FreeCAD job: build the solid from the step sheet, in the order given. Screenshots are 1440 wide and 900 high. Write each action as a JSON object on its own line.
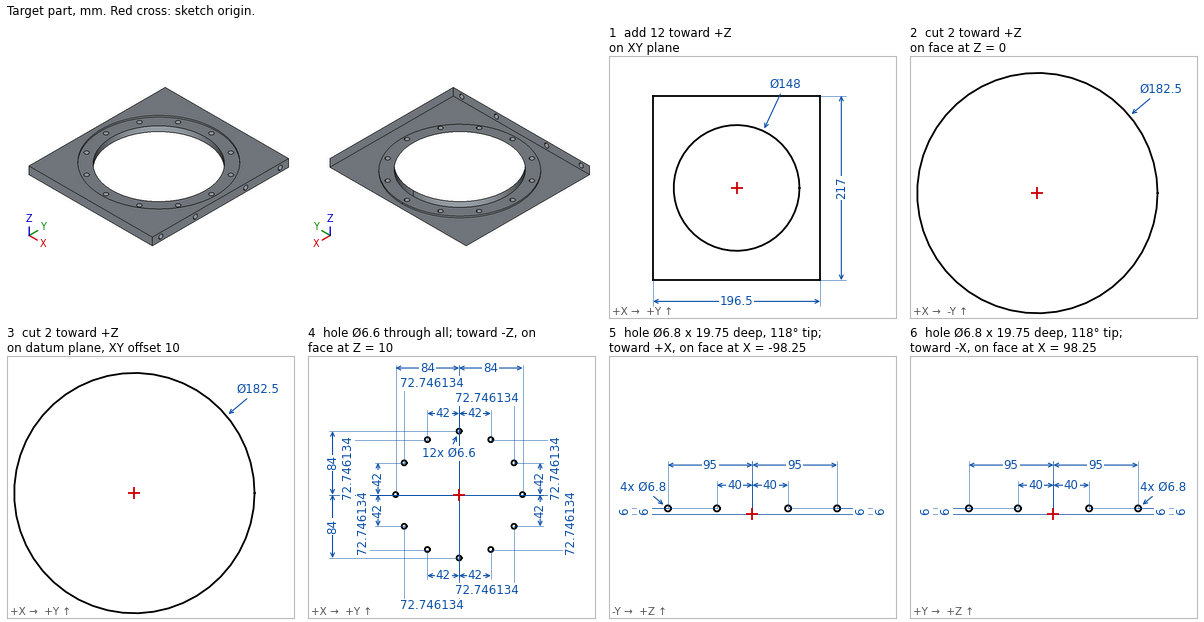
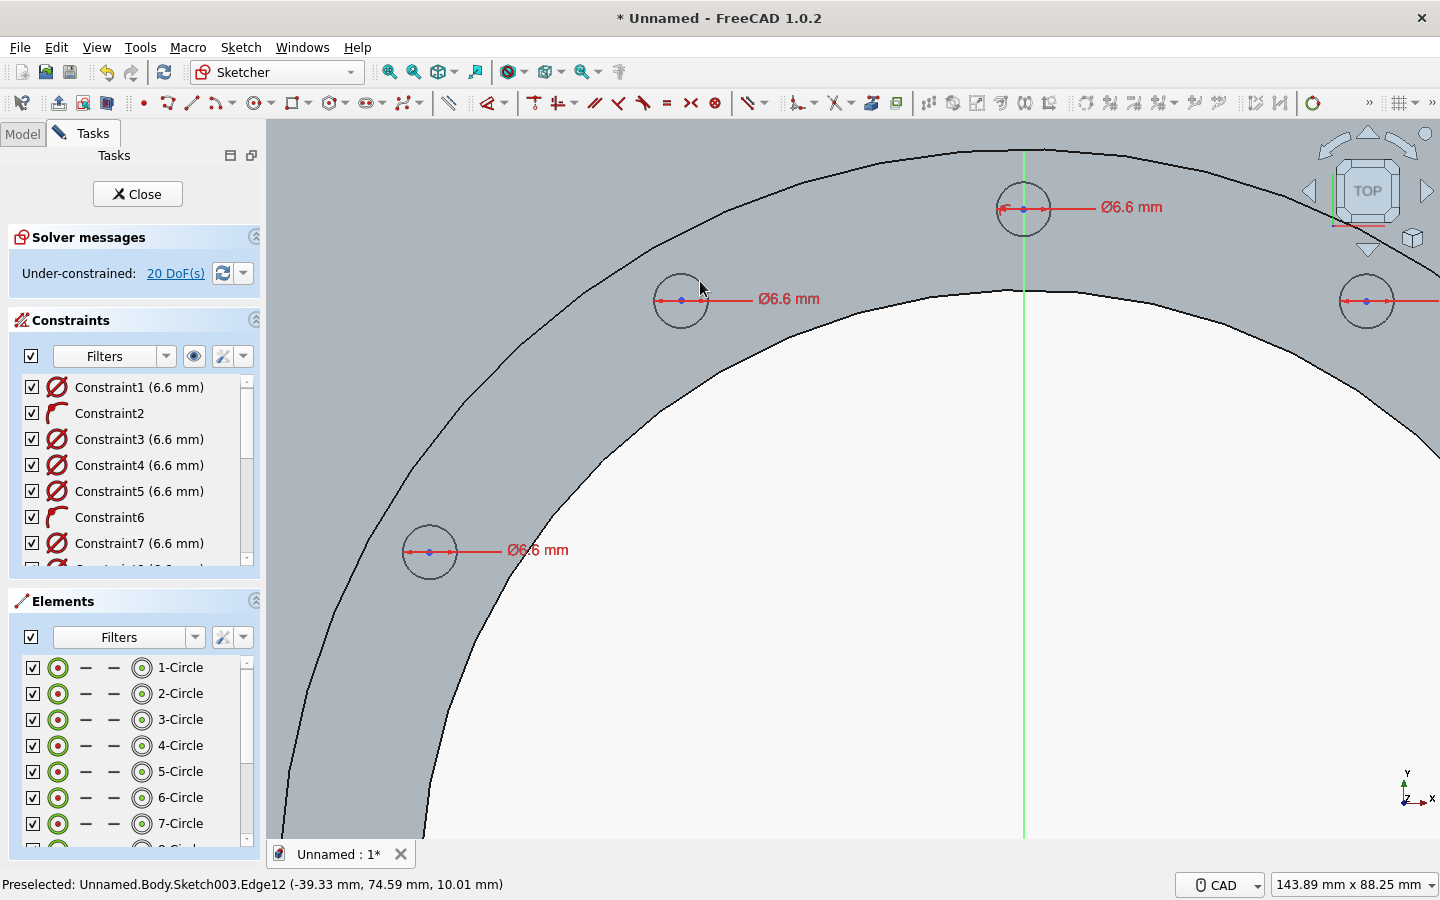
{"action": "left_click", "coordinate": [488, 104]}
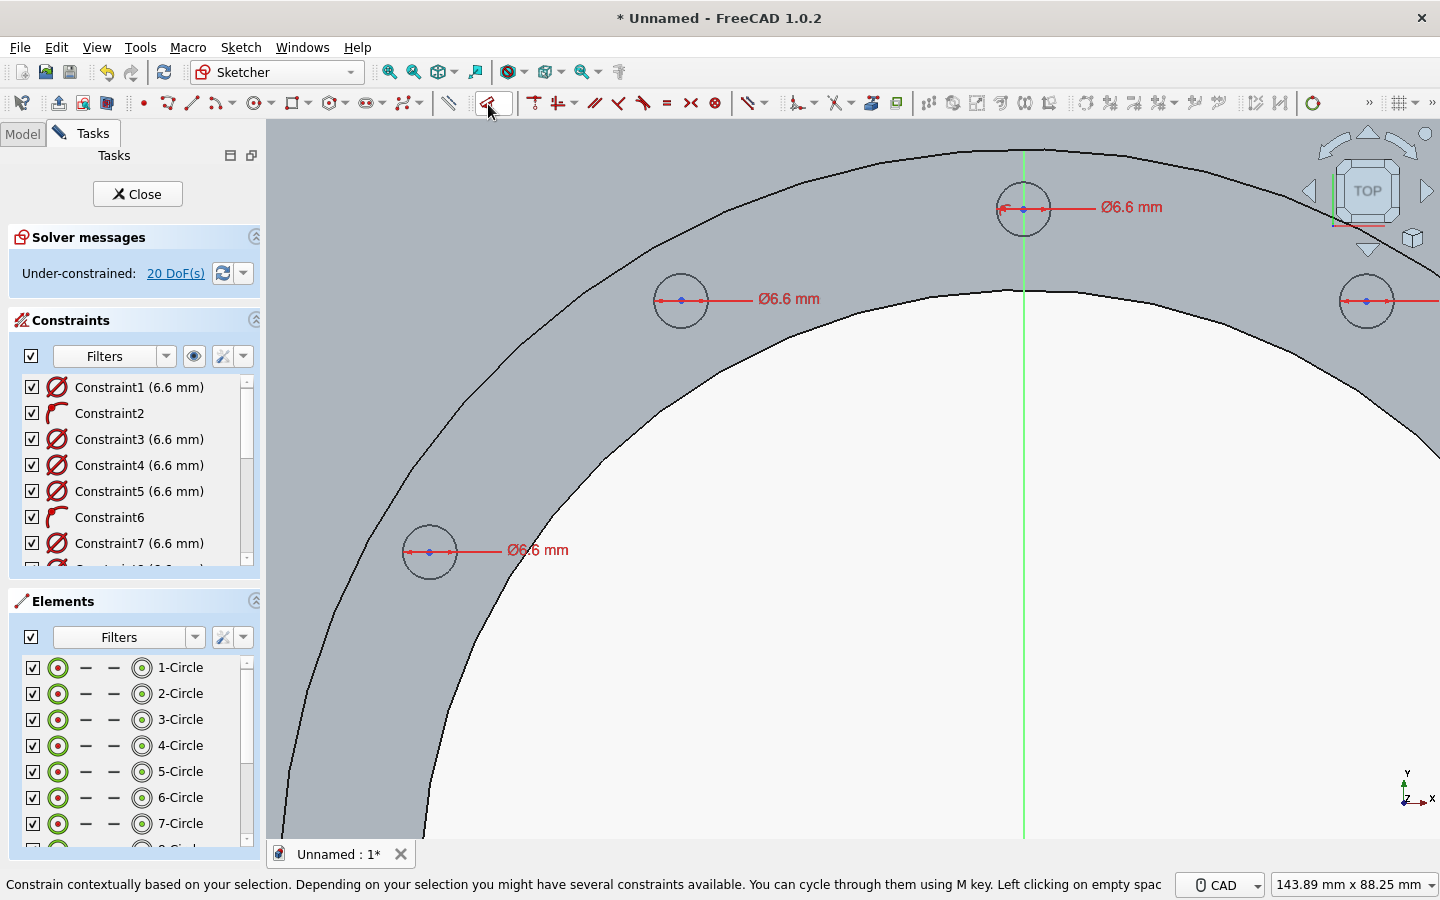
{"action": "left_click", "coordinate": [1024, 209]}
{"action": "left_click", "coordinate": [1058, 510]}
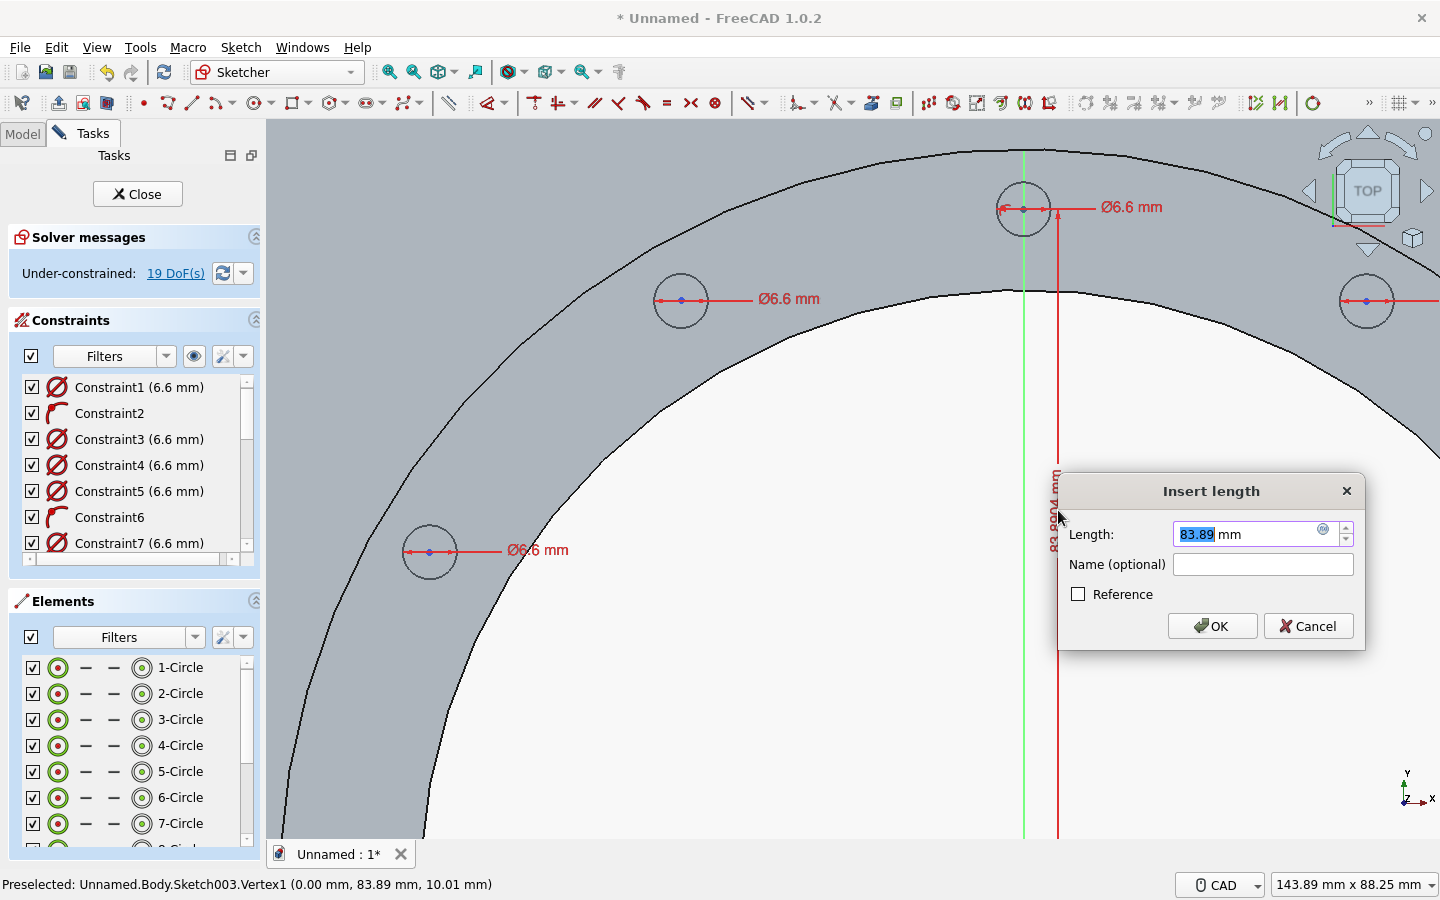
{"action": "type", "text": "84"}
{"action": "key", "text": "Return"}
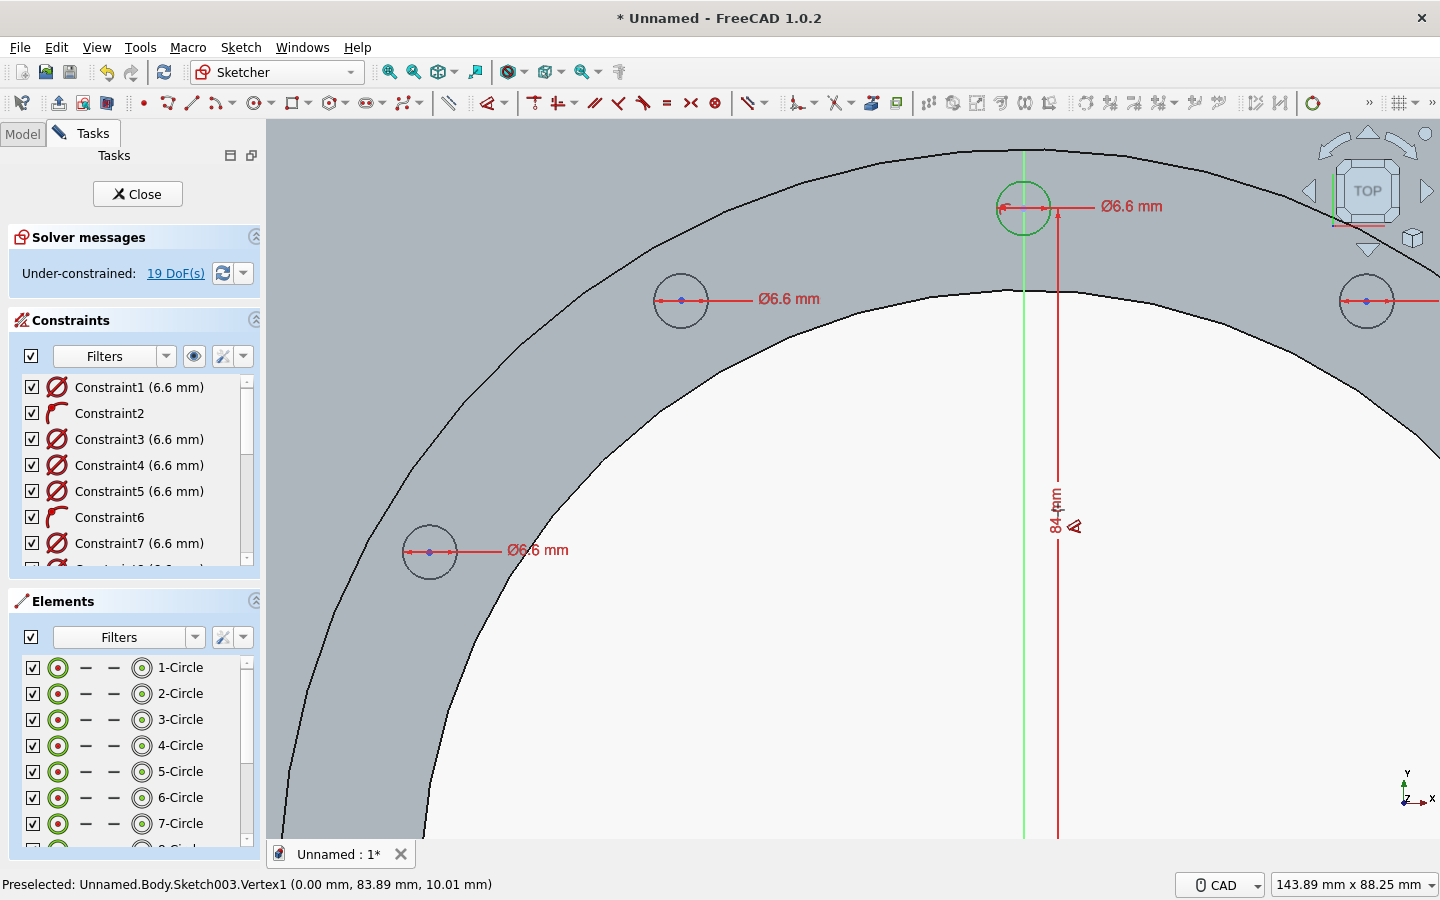
{"action": "scroll", "coordinate": [681, 300], "scroll_direction": "down", "scroll_amount": 6}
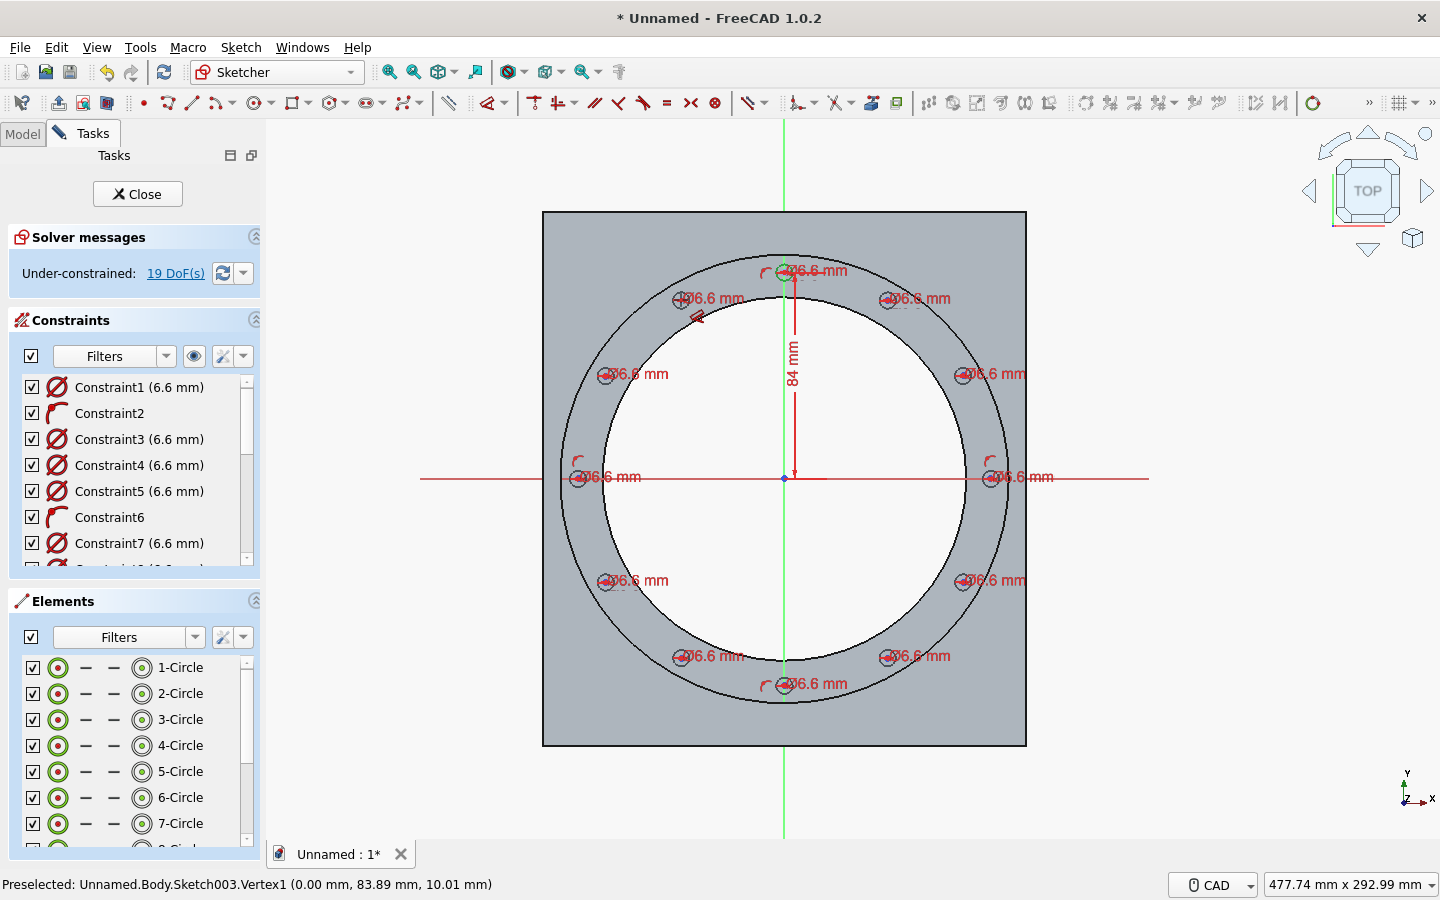
{"action": "left_click", "coordinate": [888, 301]}
{"action": "left_click", "coordinate": [836, 267]}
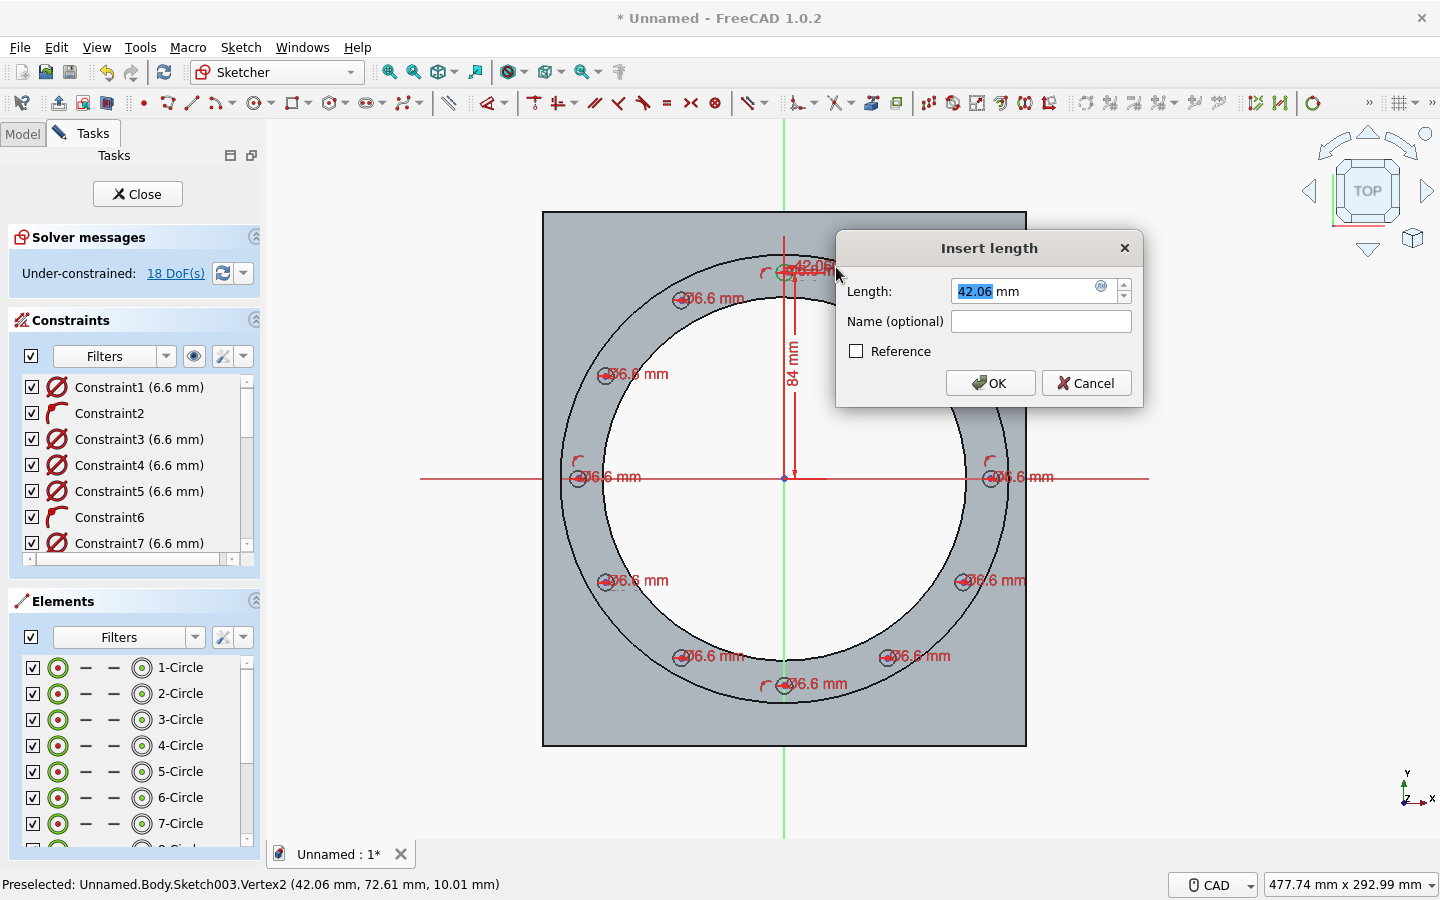
{"action": "type", "text": "42"}
{"action": "key", "text": "Return"}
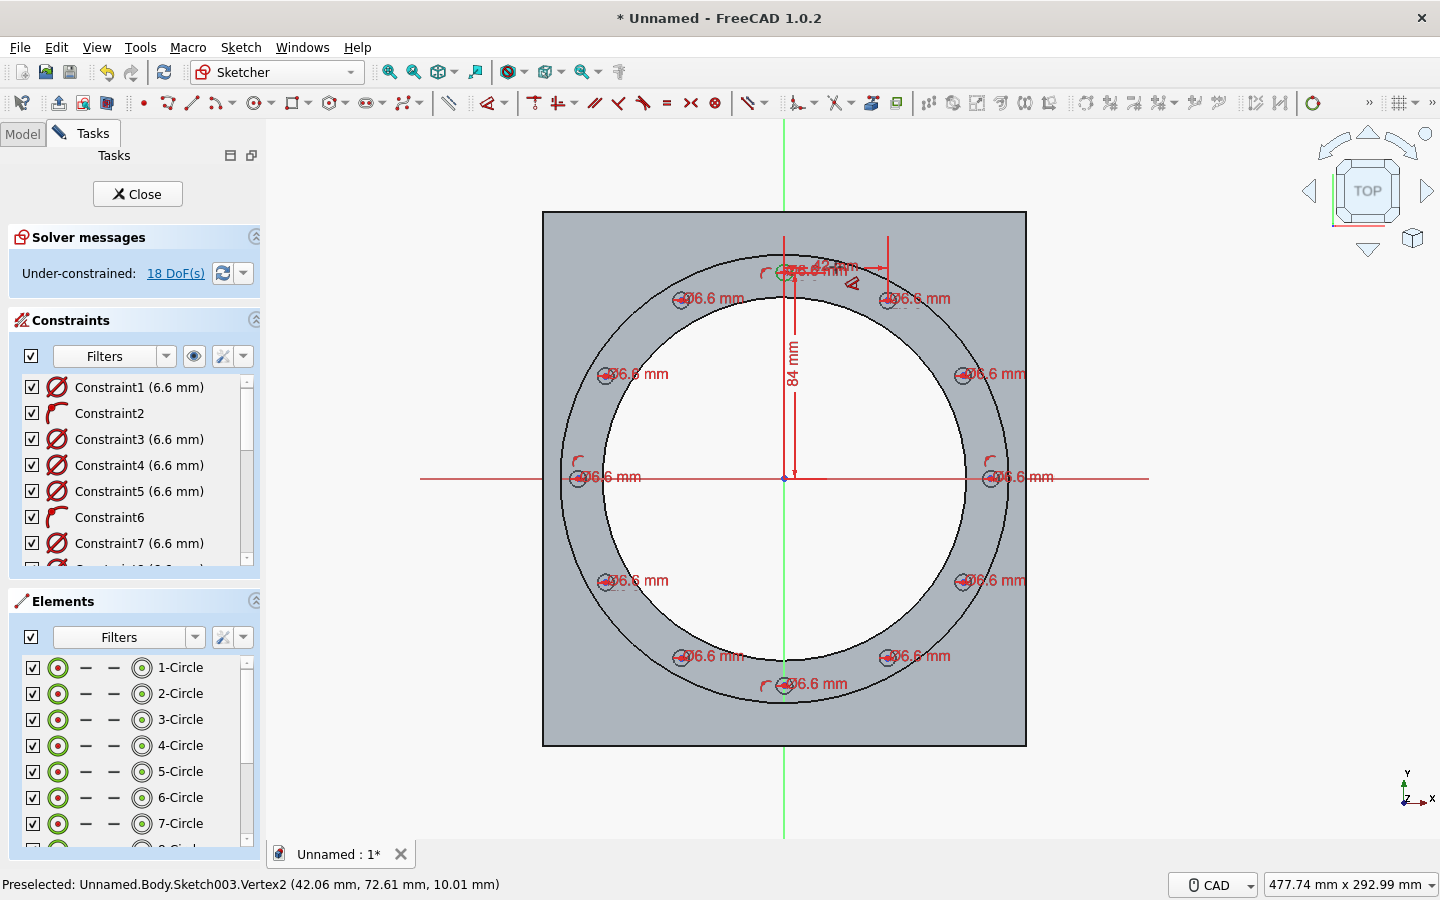
{"action": "left_click", "coordinate": [963, 376]}
{"action": "left_click", "coordinate": [997, 427]}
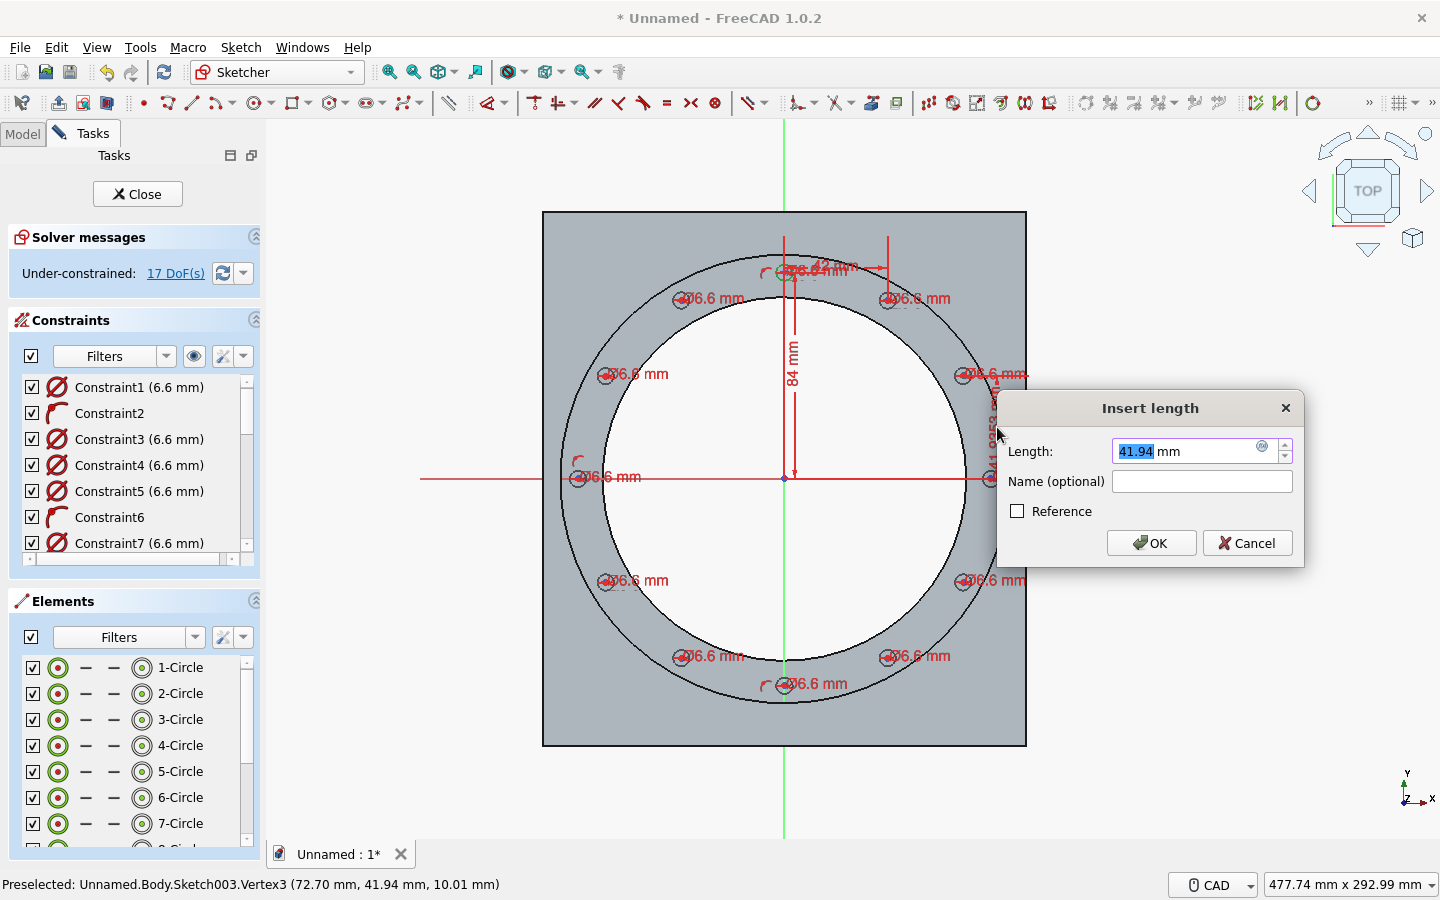
{"action": "type", "text": "42"}
{"action": "key", "text": "Return"}